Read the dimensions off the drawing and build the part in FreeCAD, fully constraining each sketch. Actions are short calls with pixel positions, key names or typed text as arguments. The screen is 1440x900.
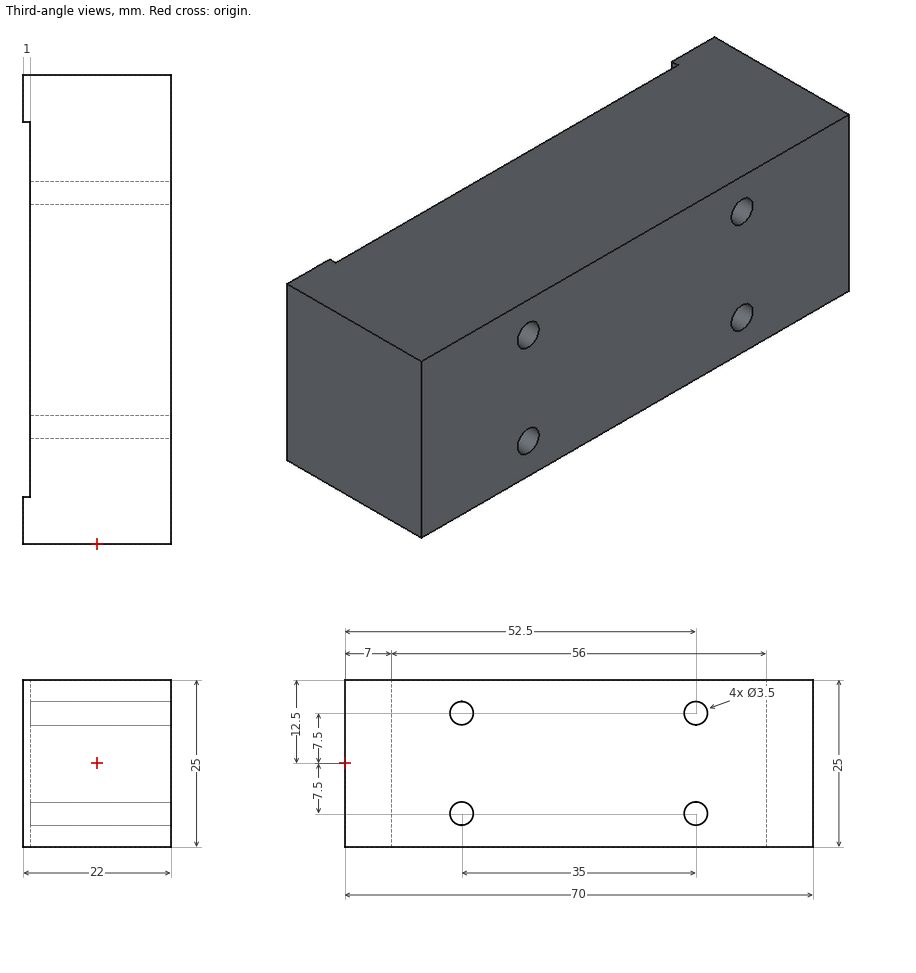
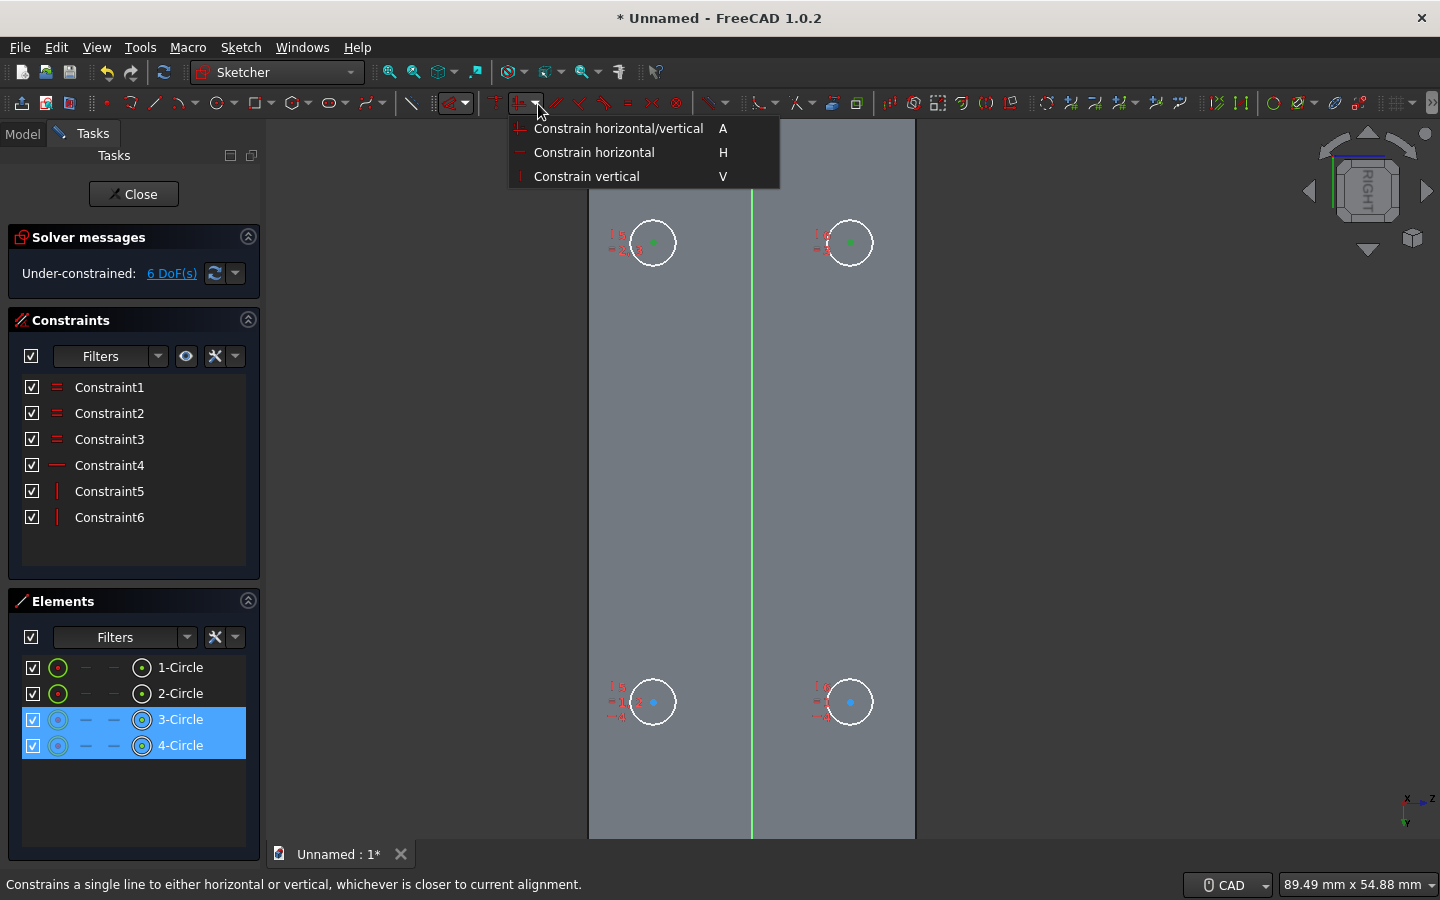
click(644, 152)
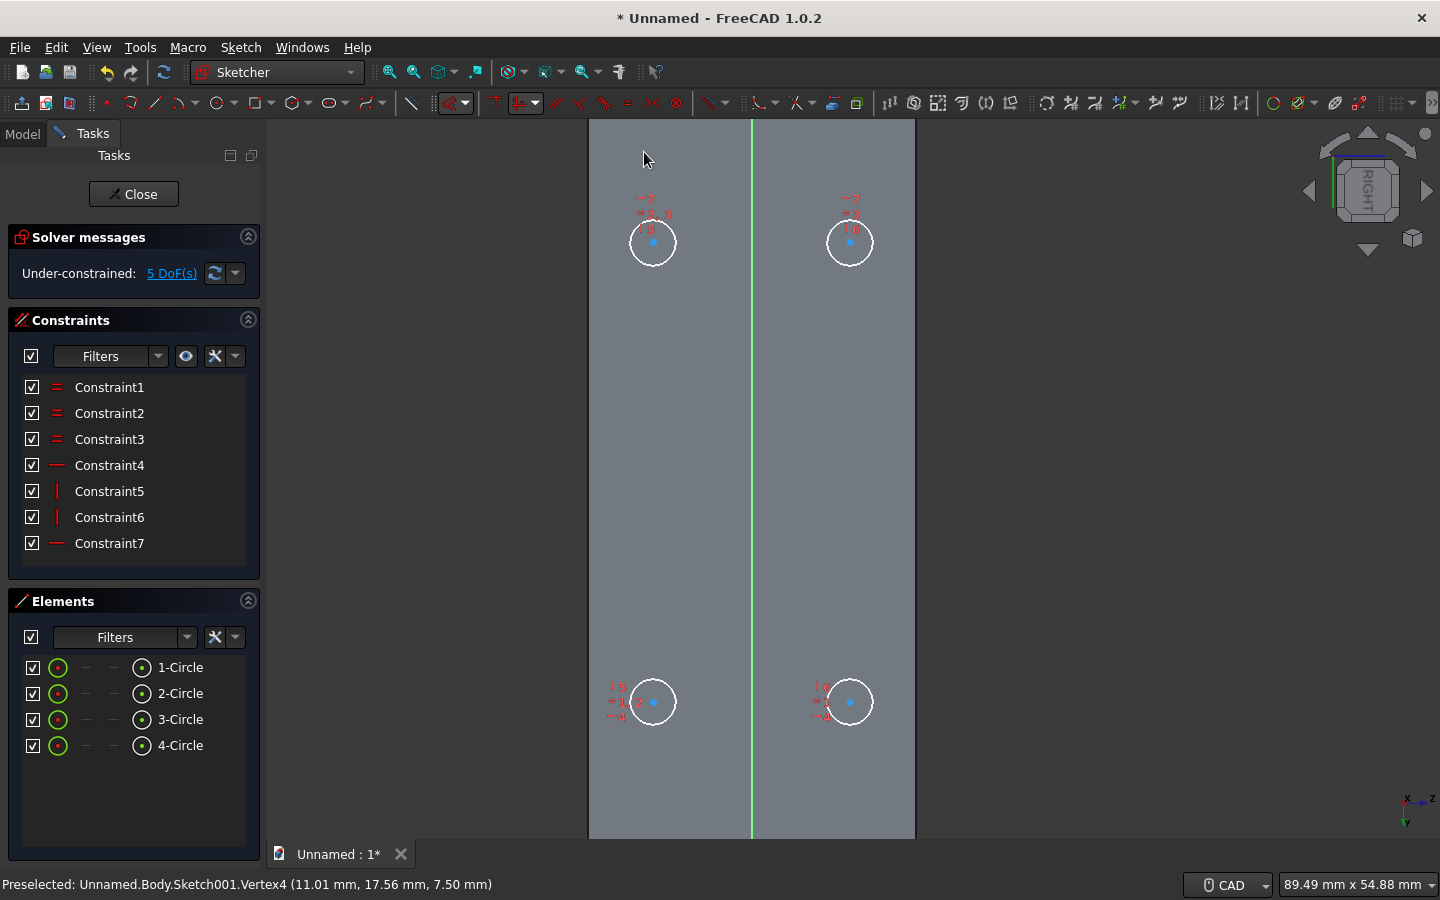
click(866, 686)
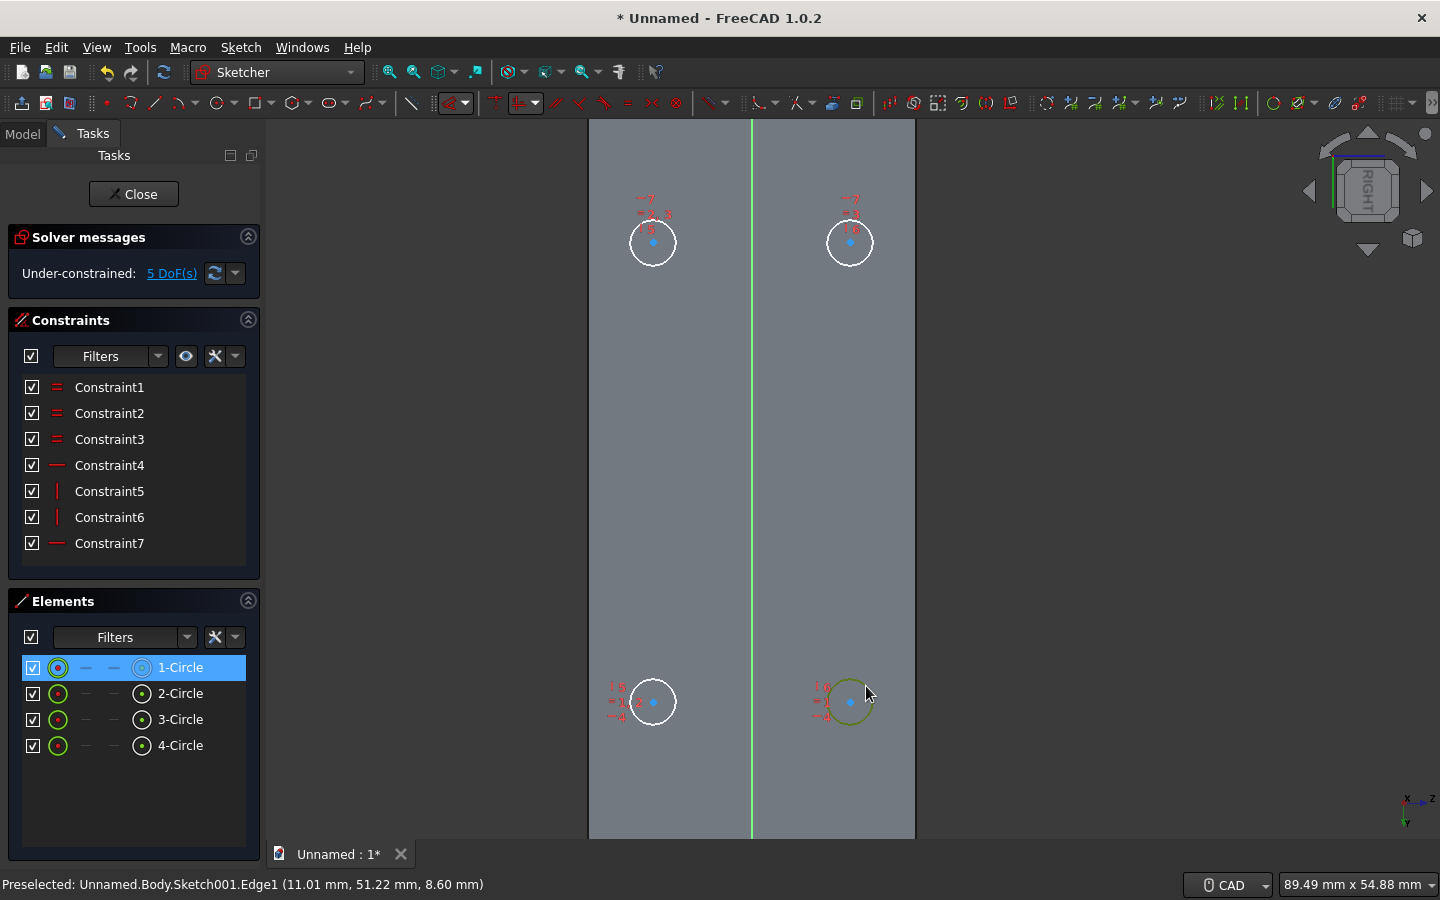
key(k)
key(o)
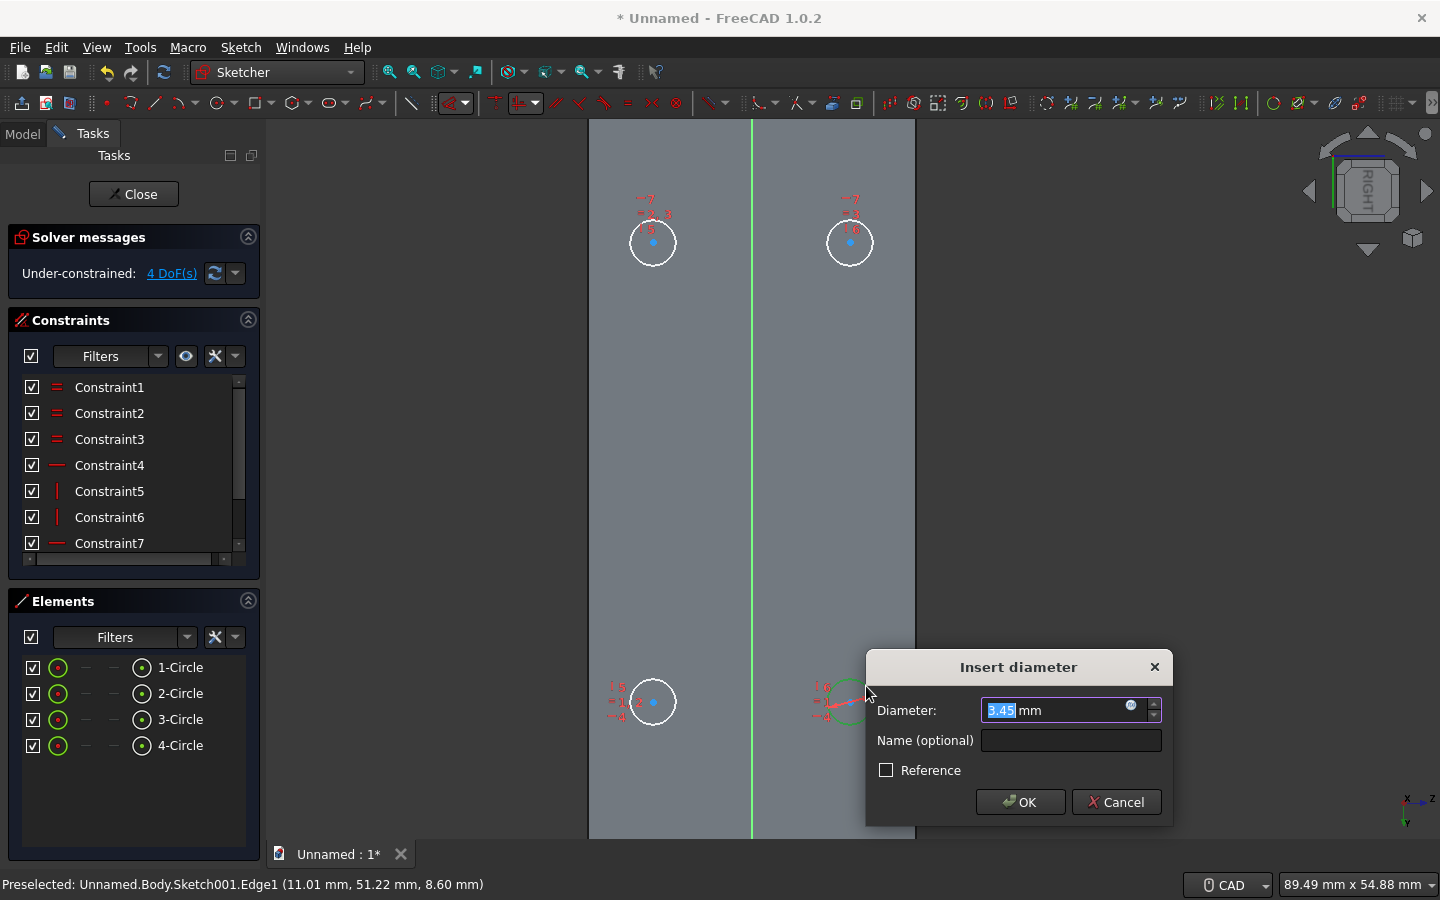
text(3.5)
key(Return)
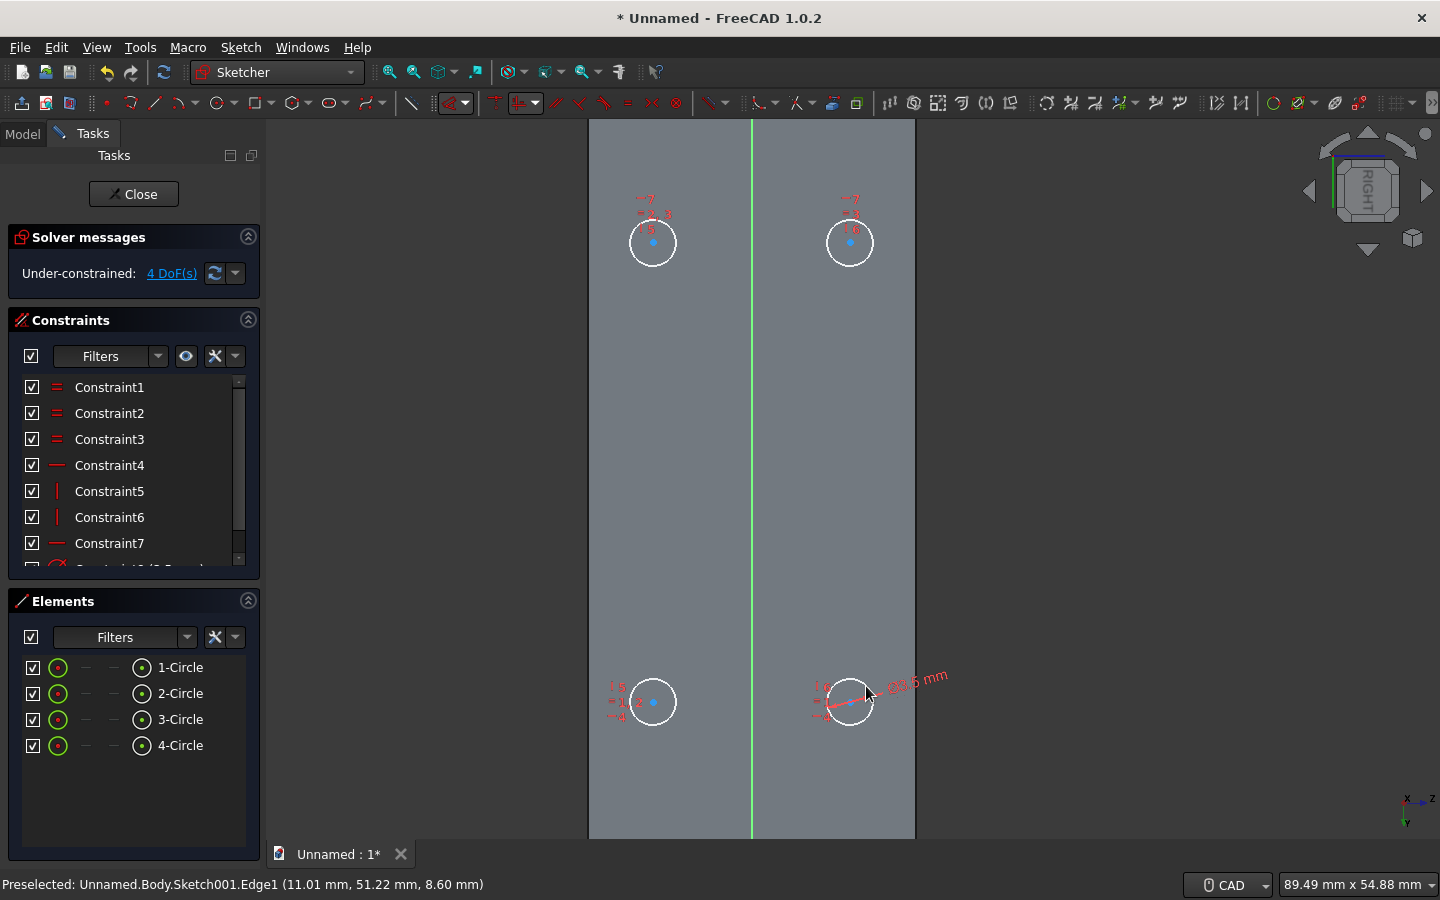
click(850, 702)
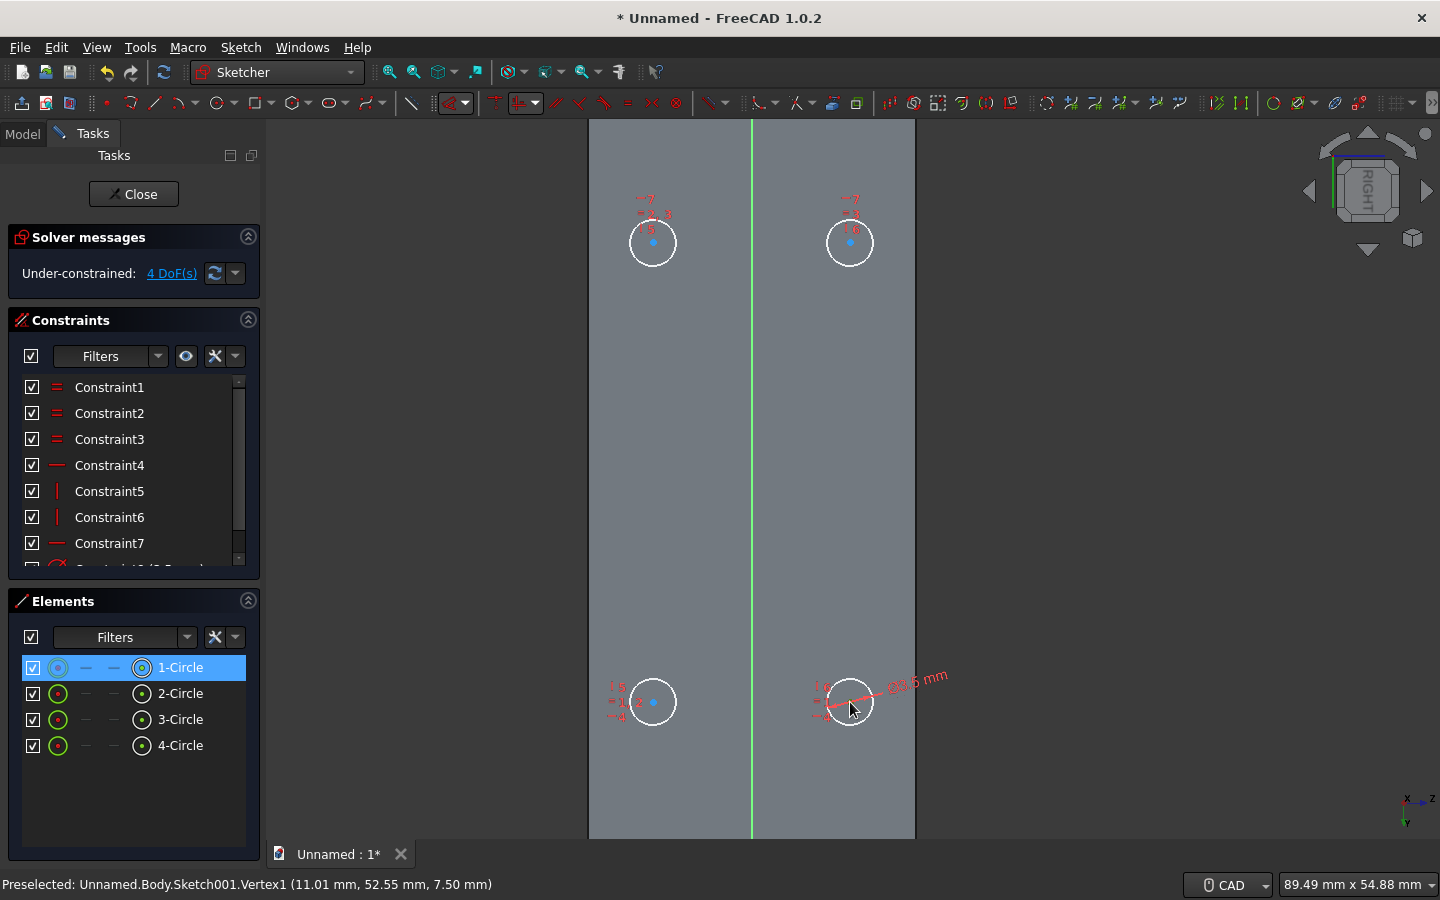
key(l)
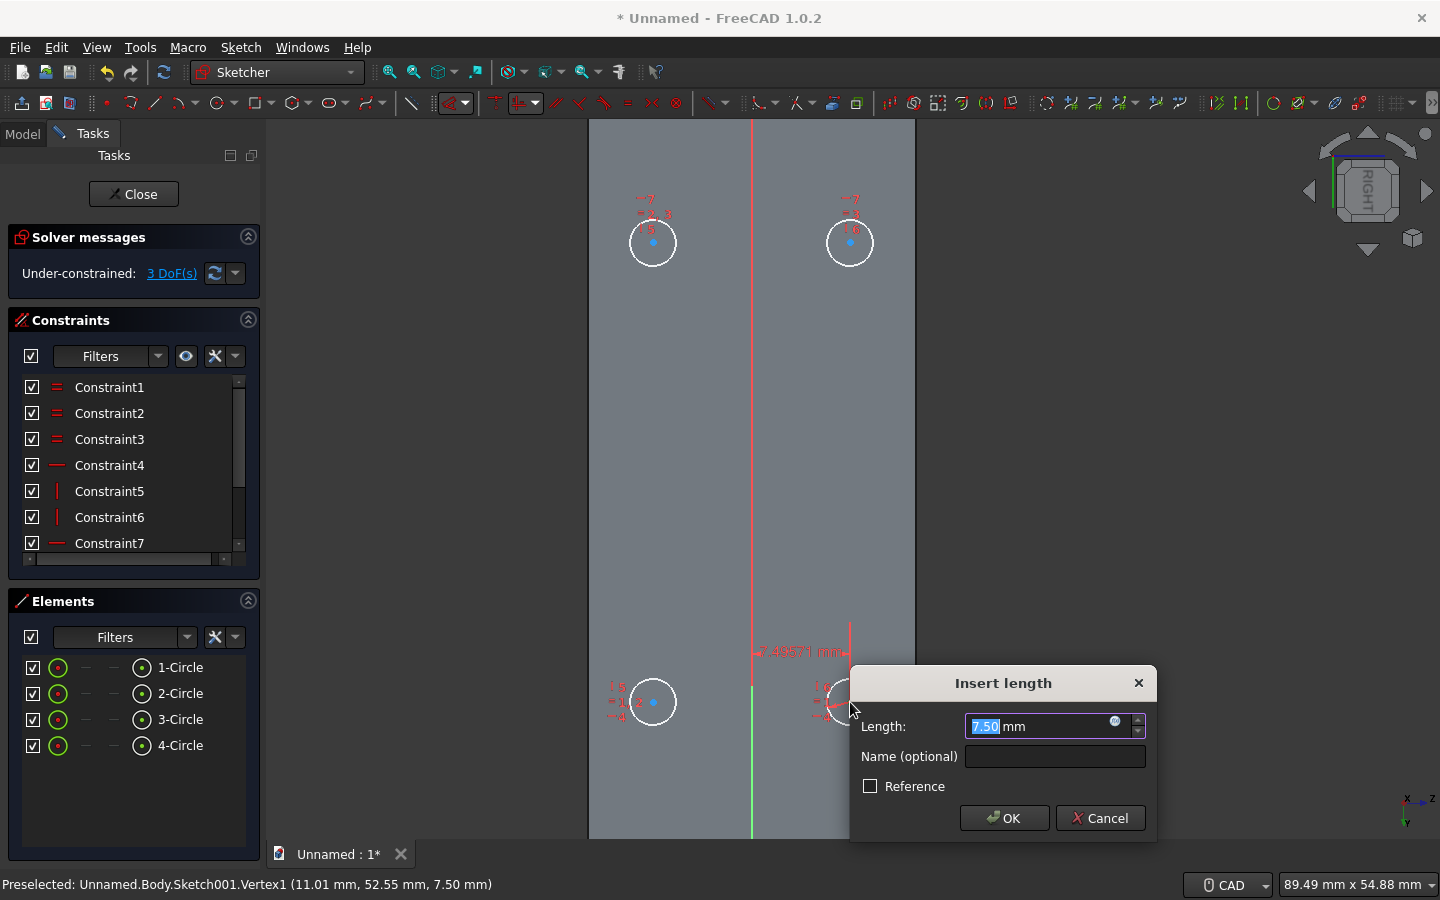
text(7.5)
key(Return)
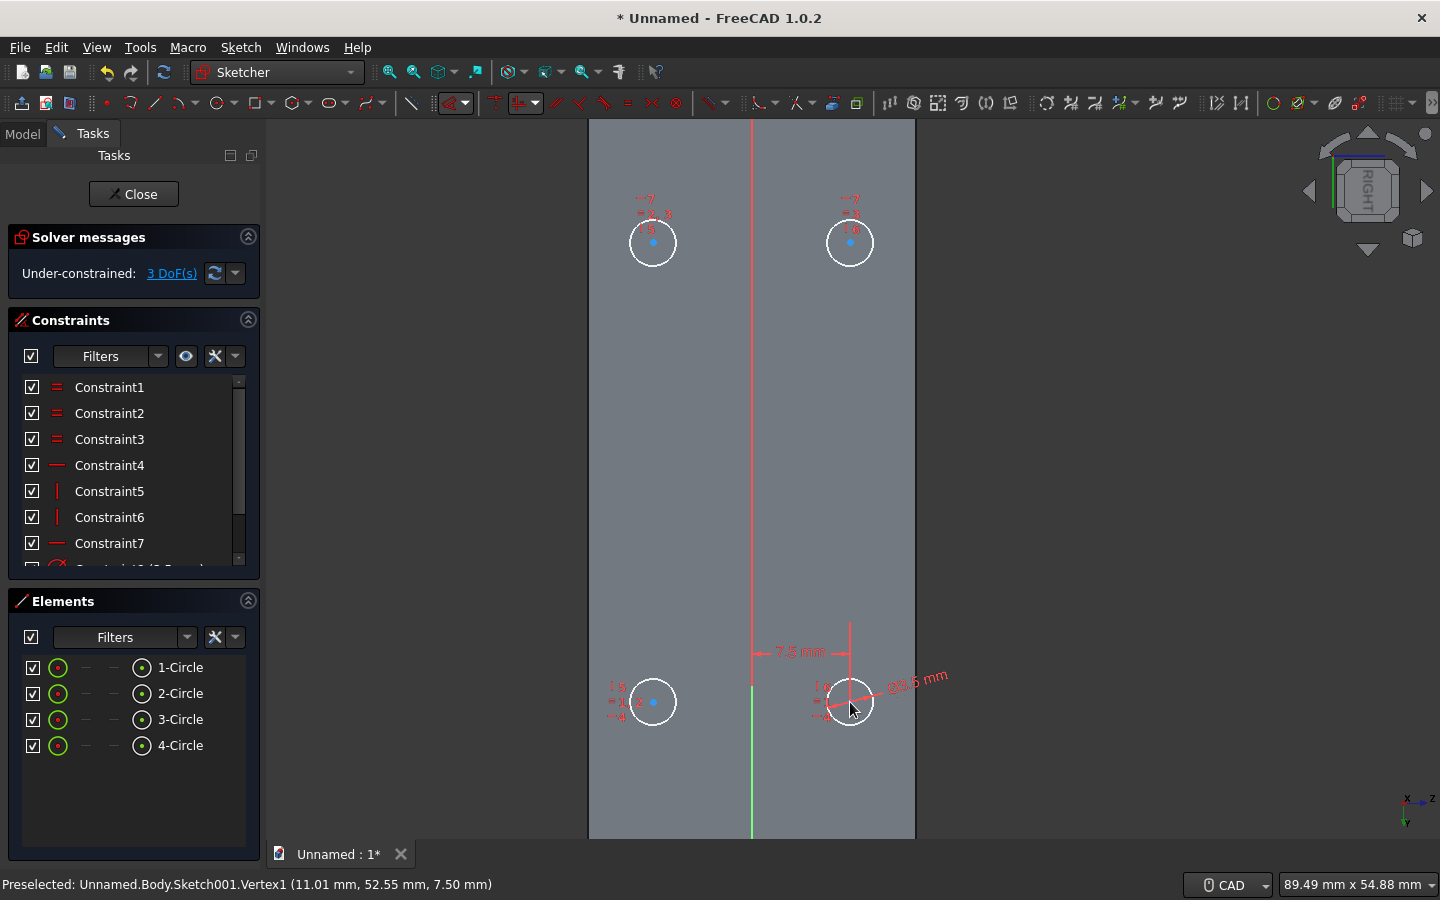
click(653, 702)